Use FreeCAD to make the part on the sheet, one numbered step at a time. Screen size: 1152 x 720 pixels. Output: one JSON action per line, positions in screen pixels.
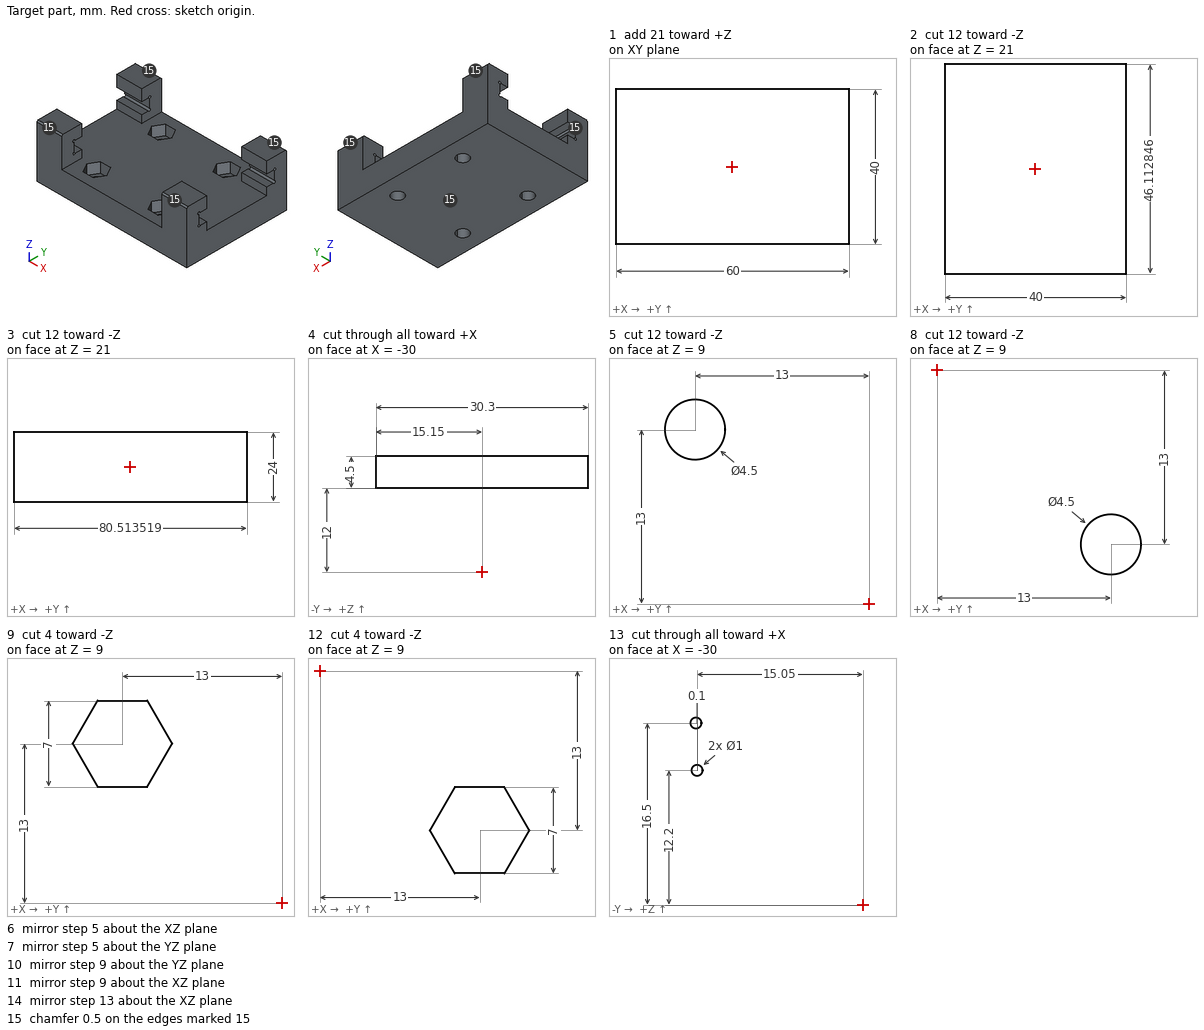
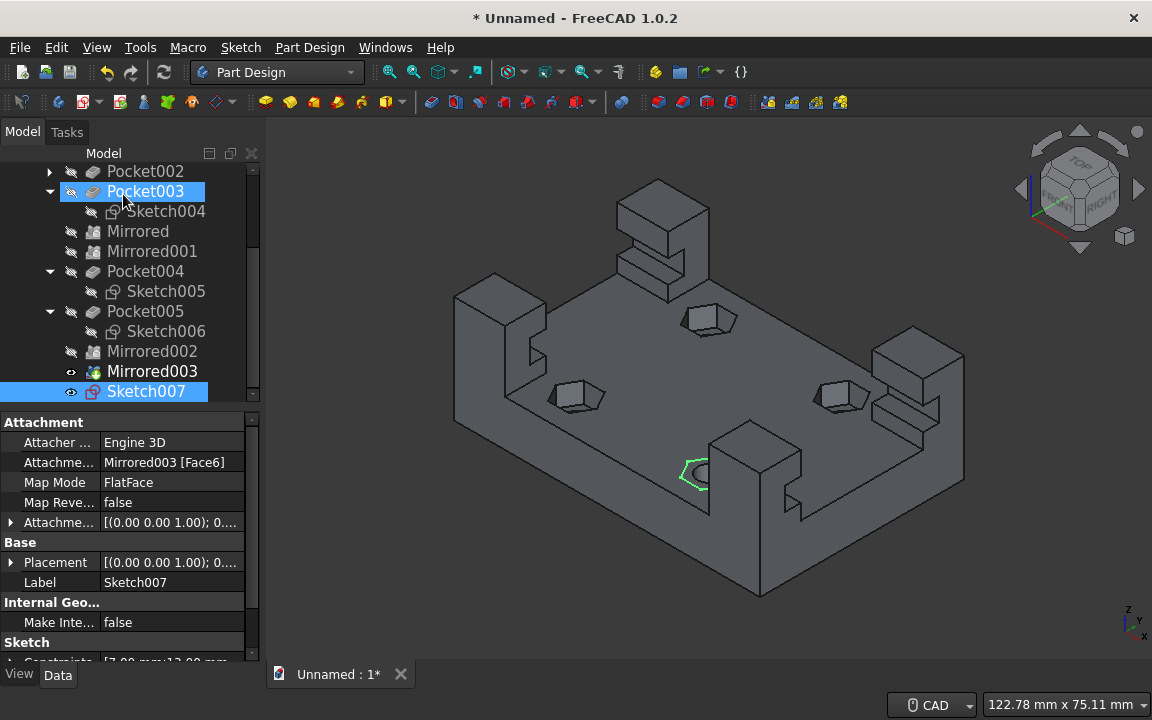
{"action": "left_click", "coordinate": [432, 102]}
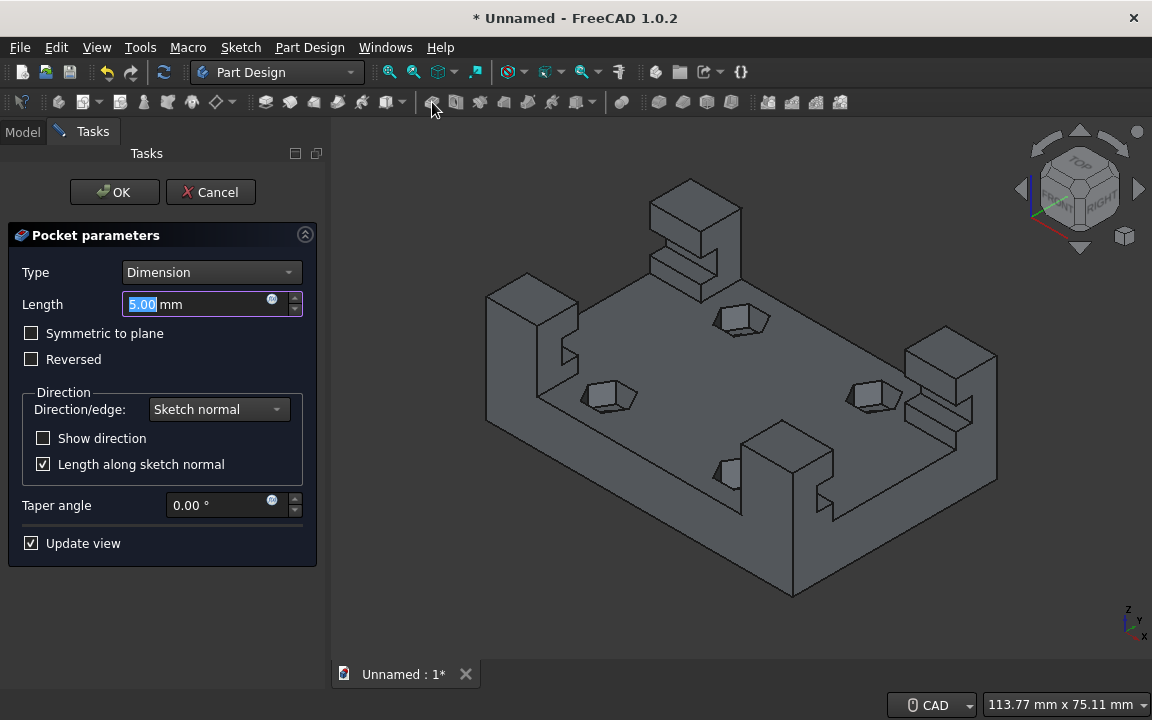
{"action": "type", "text": "4"}
{"action": "key", "text": "Tab"}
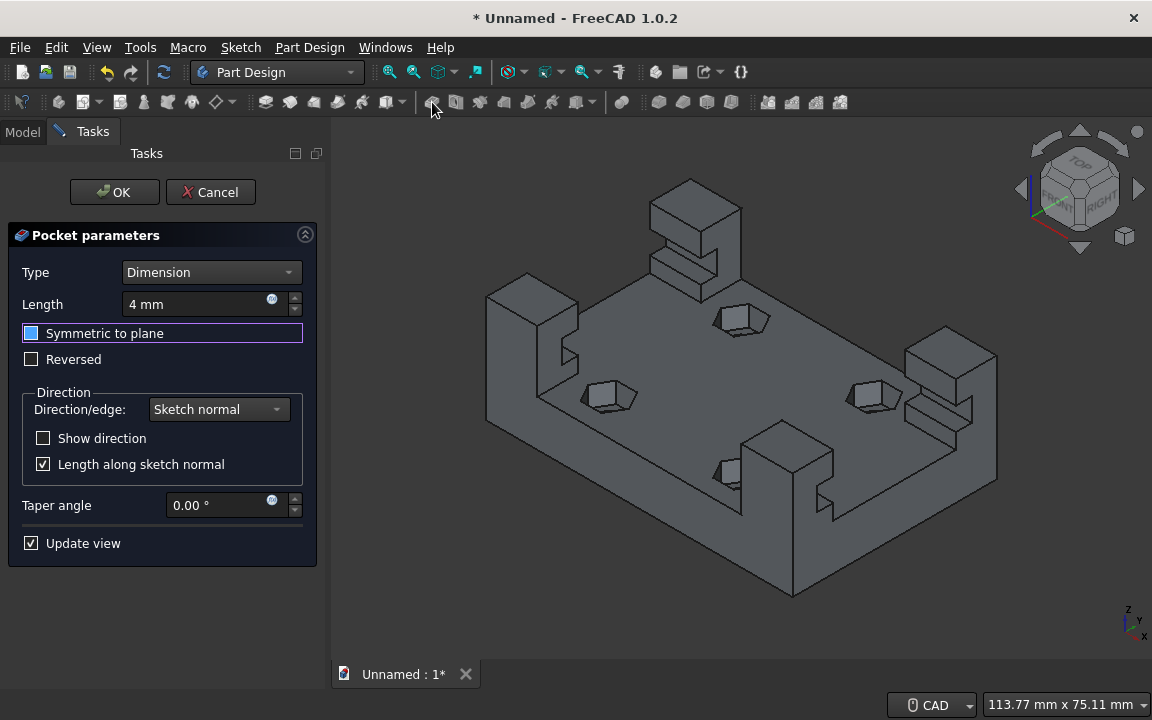
{"action": "left_click", "coordinate": [115, 192]}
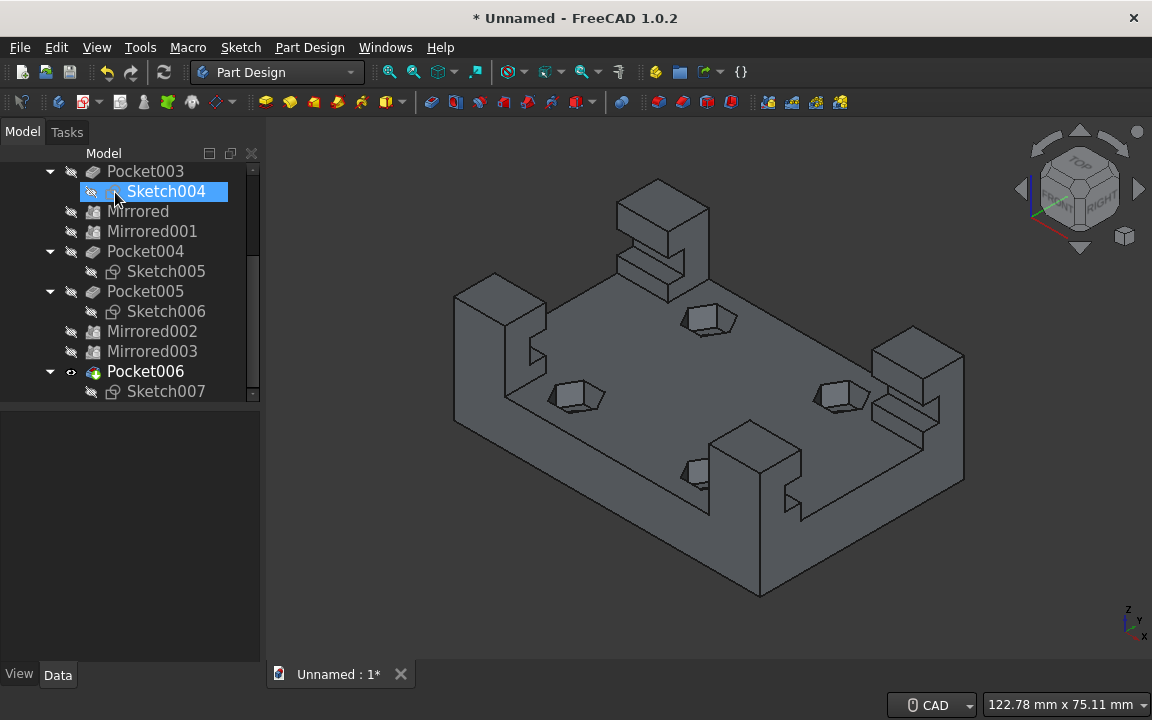
{"action": "key", "text": "6"}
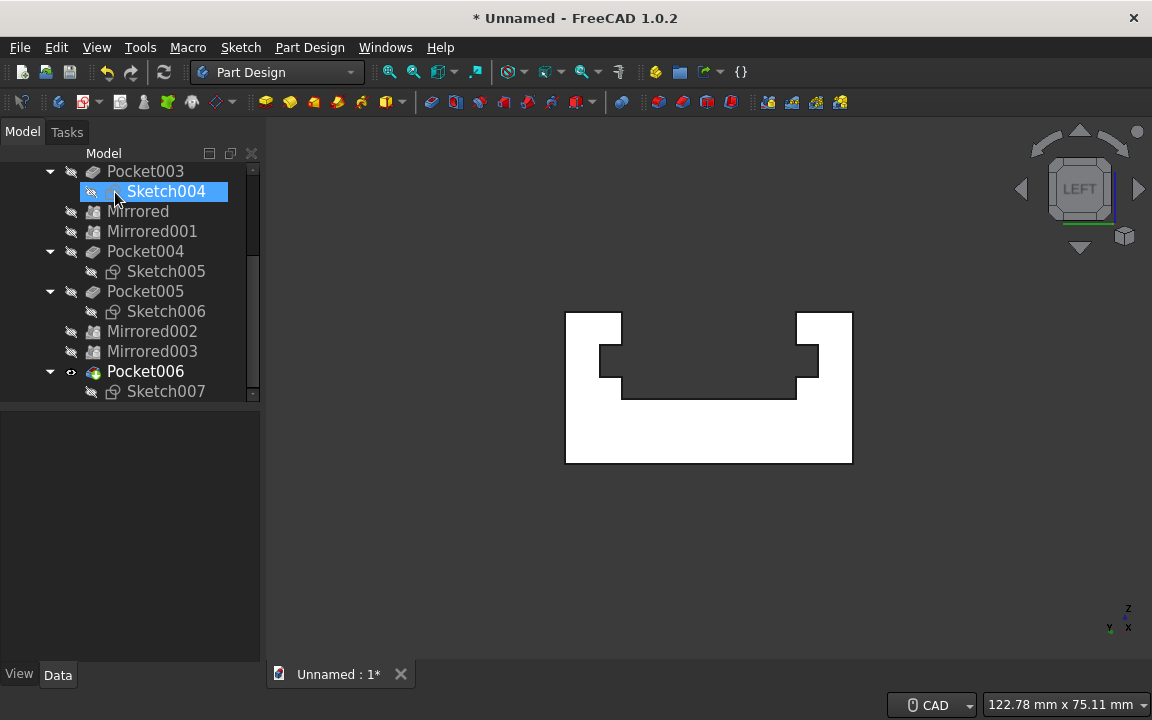
{"action": "left_click", "coordinate": [390, 72]}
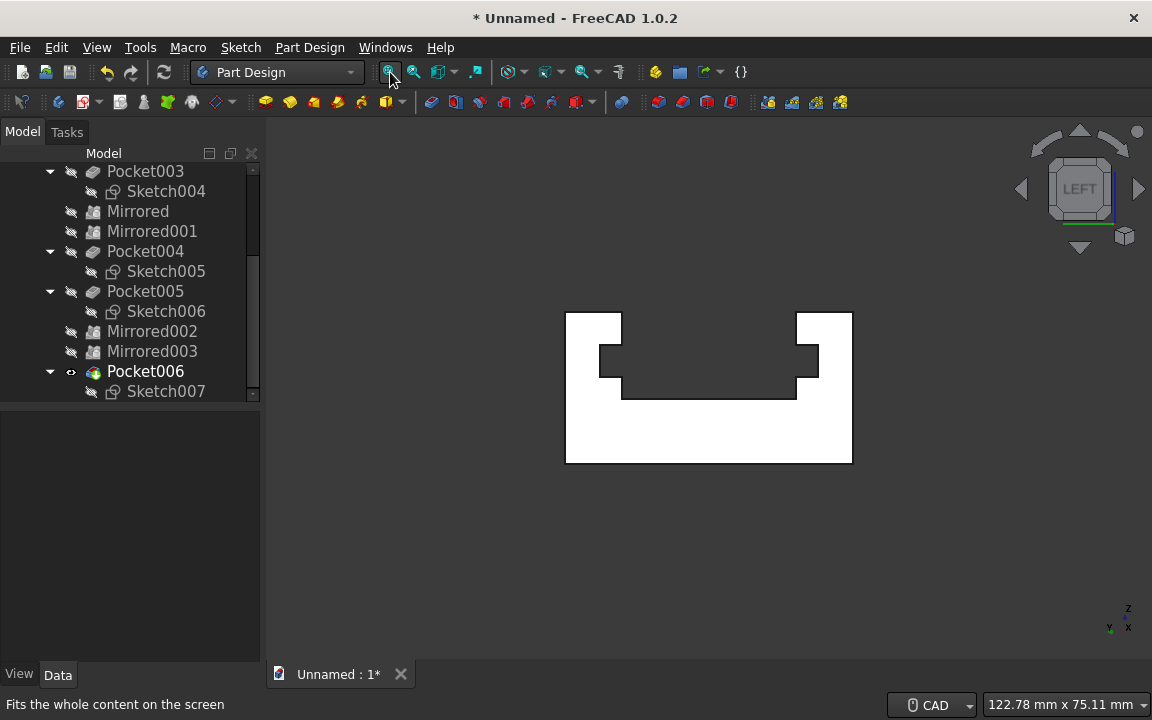
{"action": "left_click", "coordinate": [627, 430]}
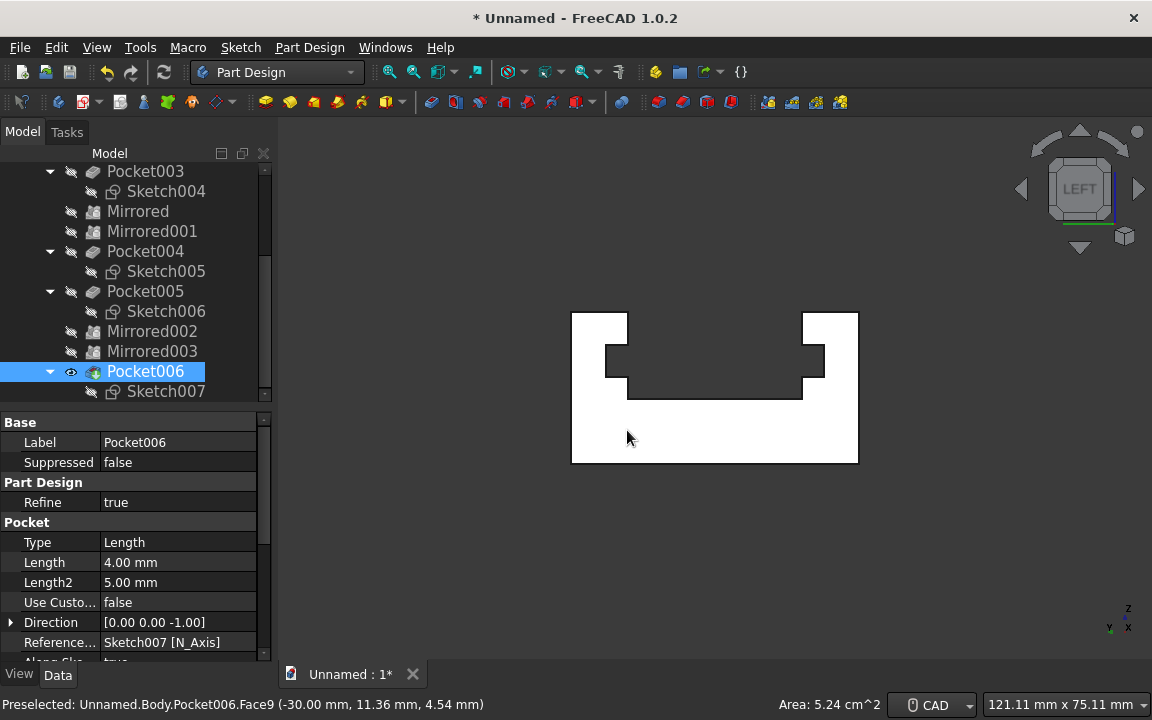
{"action": "left_click", "coordinate": [84, 102]}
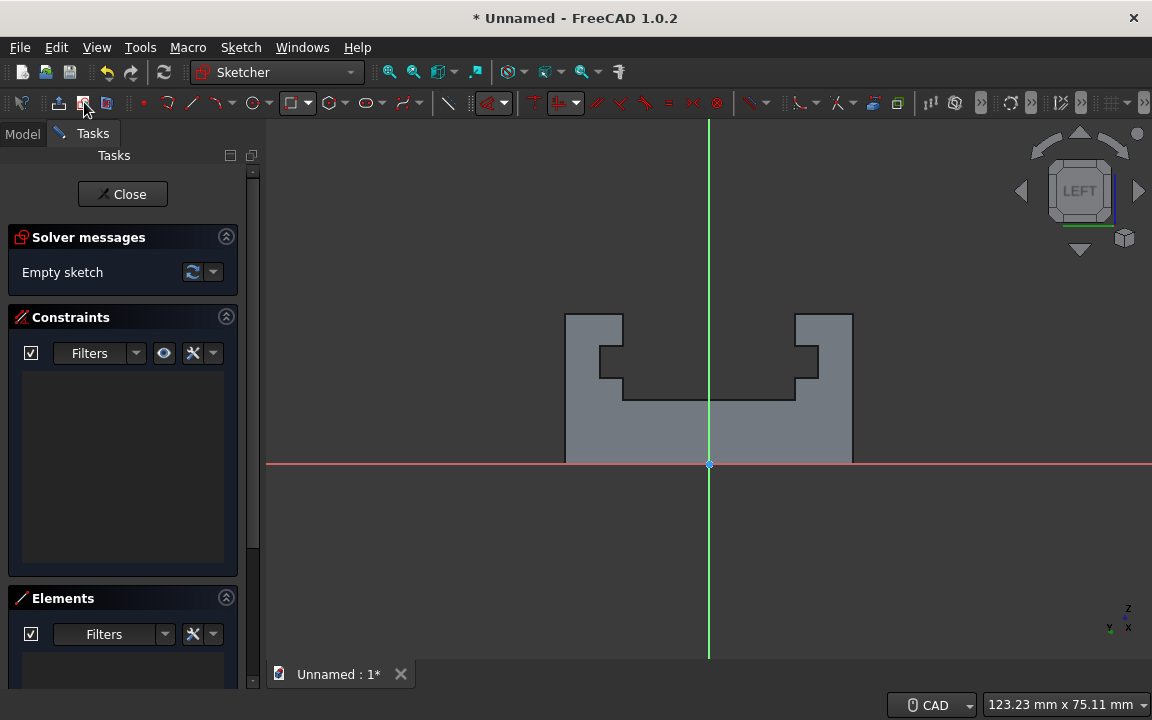
{"action": "scroll", "coordinate": [595, 358], "scroll_direction": "up", "scroll_amount": 11}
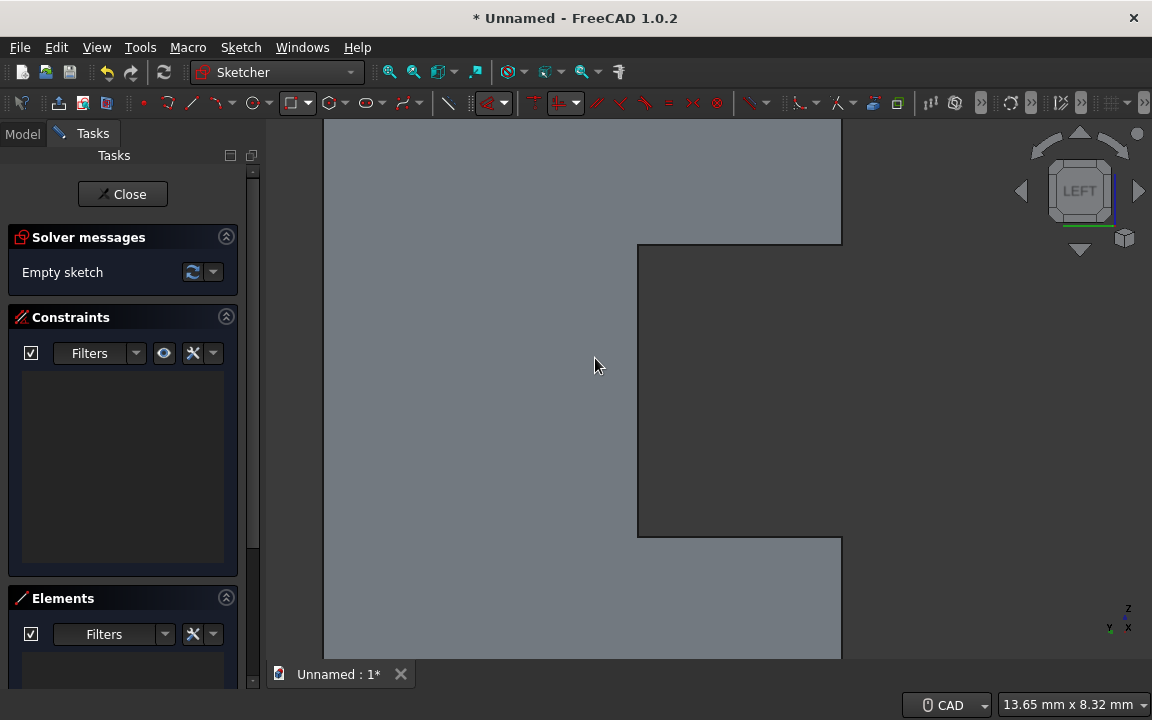
{"action": "left_click", "coordinate": [254, 104]}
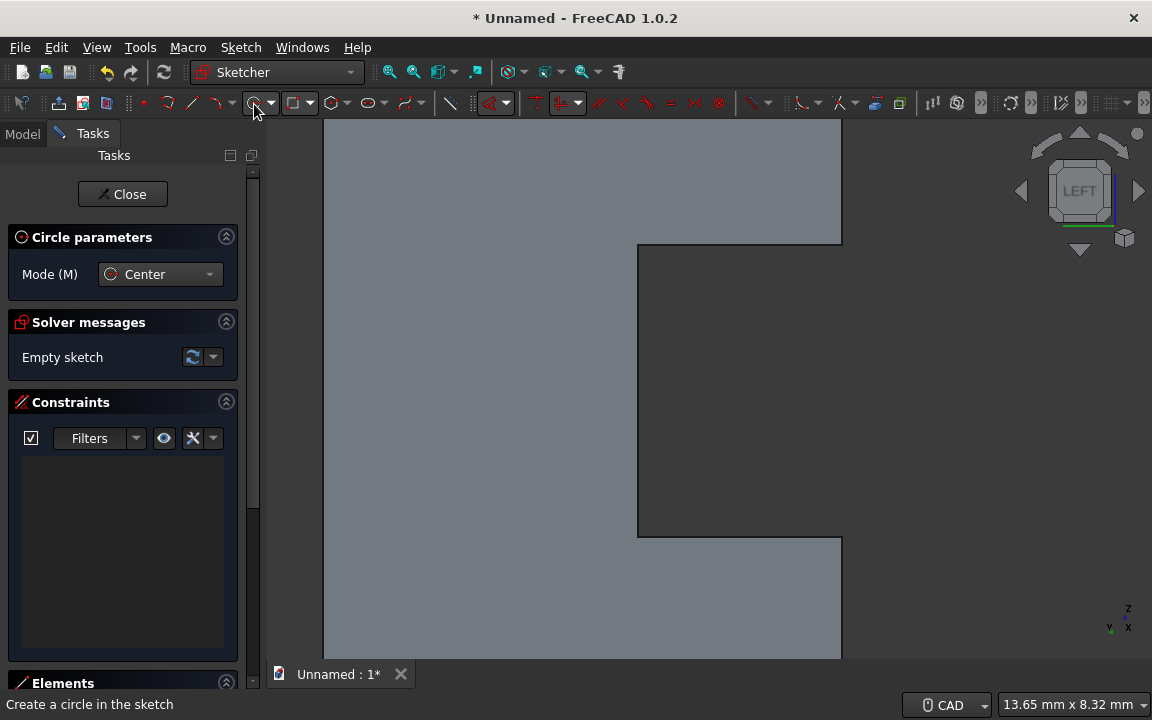
{"action": "left_click", "coordinate": [644, 524]}
{"action": "left_click", "coordinate": [667, 501]}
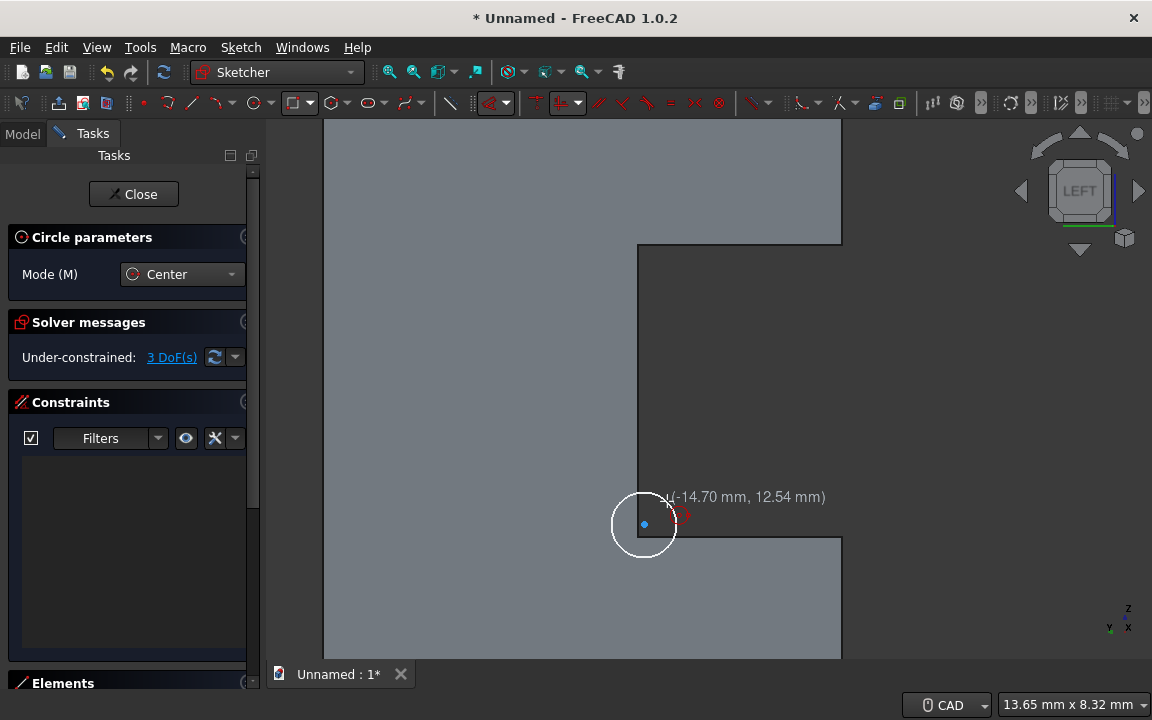
{"action": "left_click", "coordinate": [638, 245]}
{"action": "left_click", "coordinate": [661, 222]}
{"action": "key", "text": "Escape"}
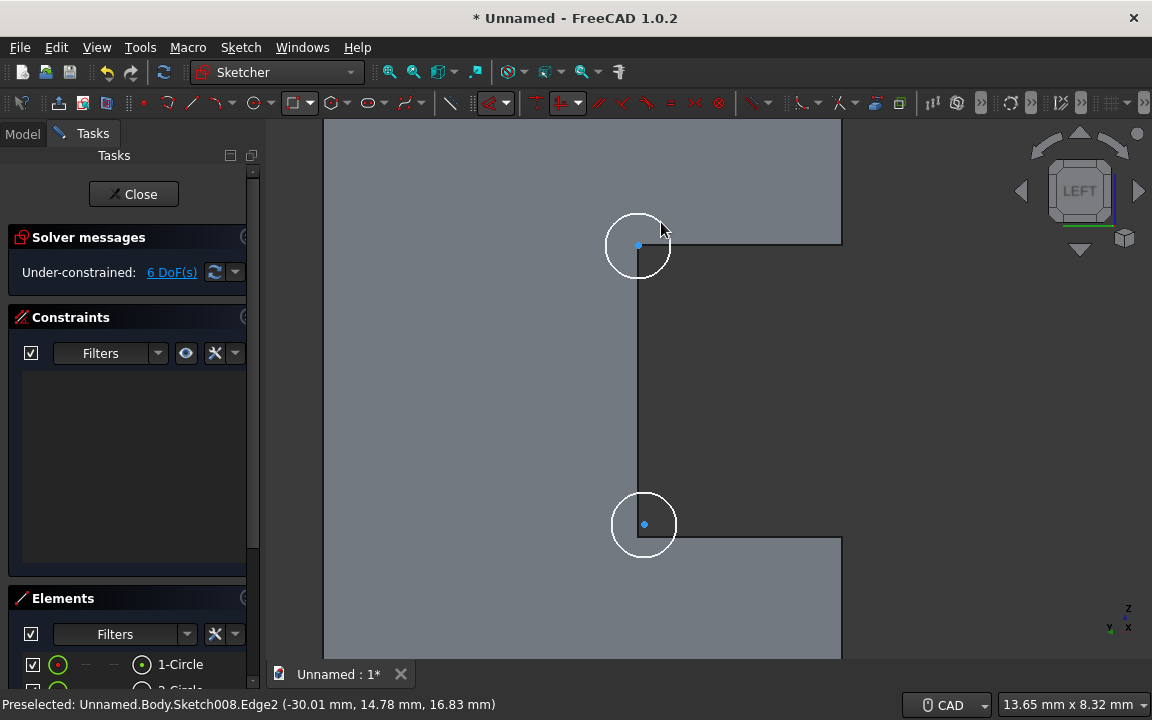
{"action": "left_click", "coordinate": [667, 502]}